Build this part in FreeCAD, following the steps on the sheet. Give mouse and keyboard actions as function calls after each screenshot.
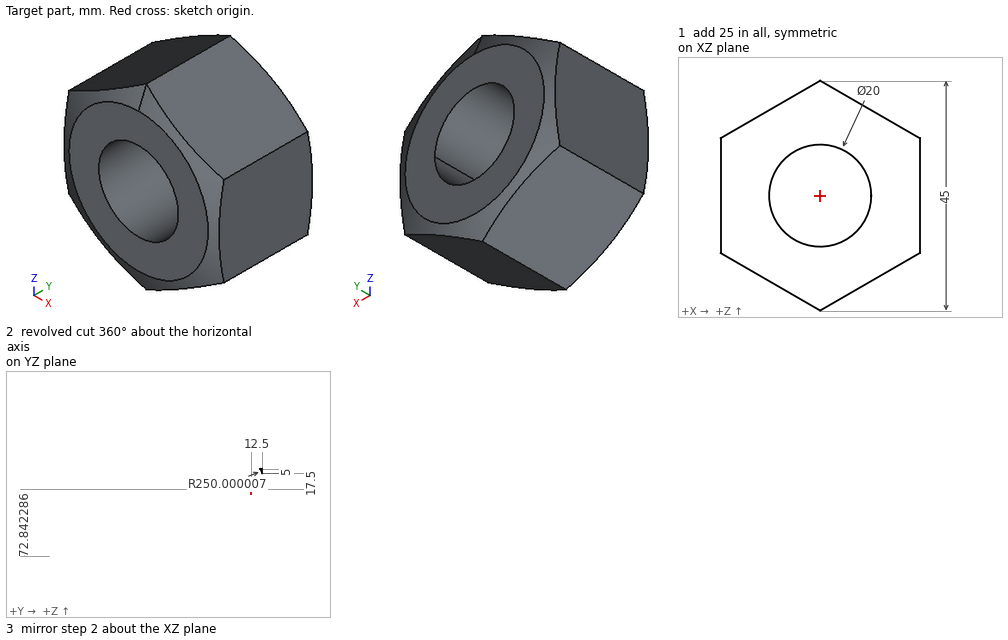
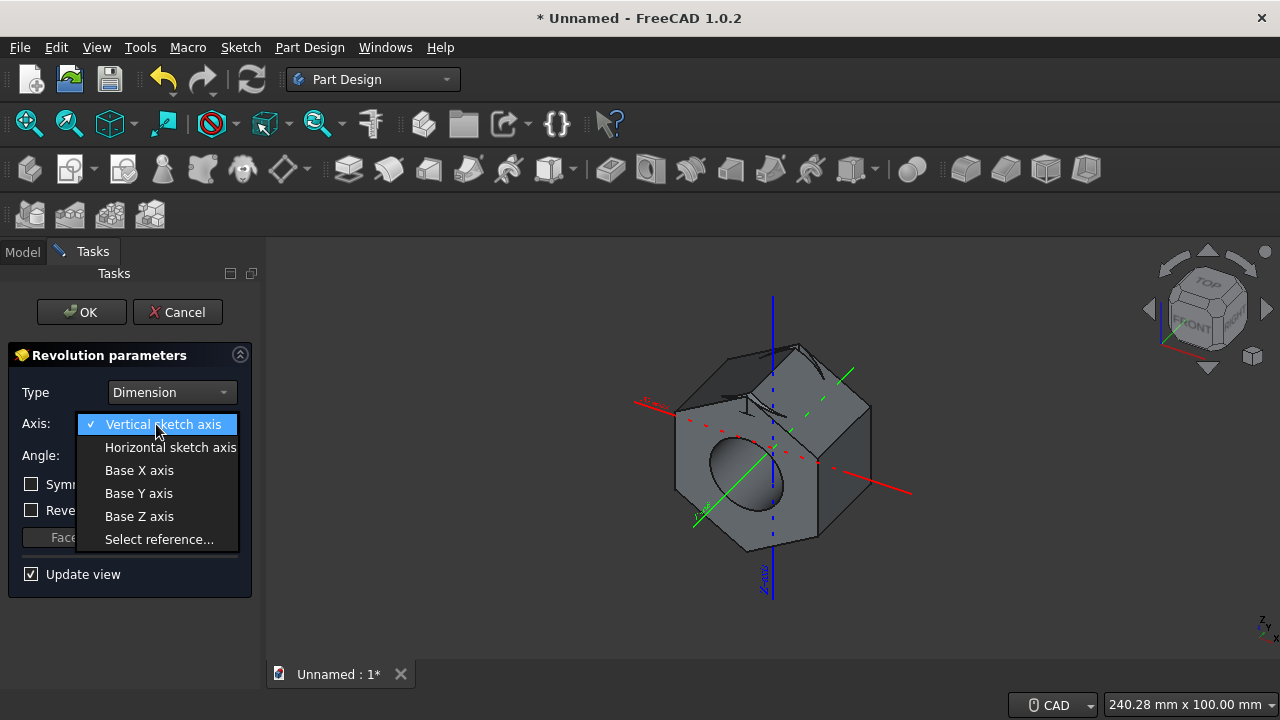
click(156, 448)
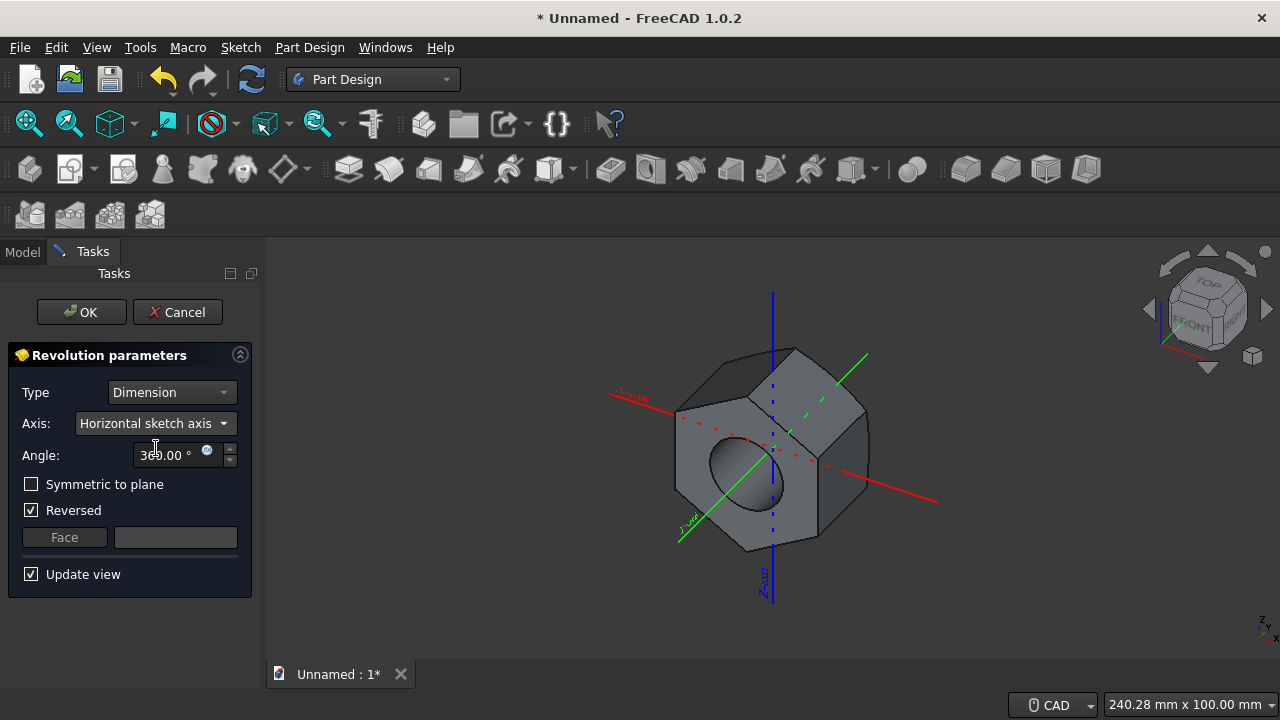
click(82, 312)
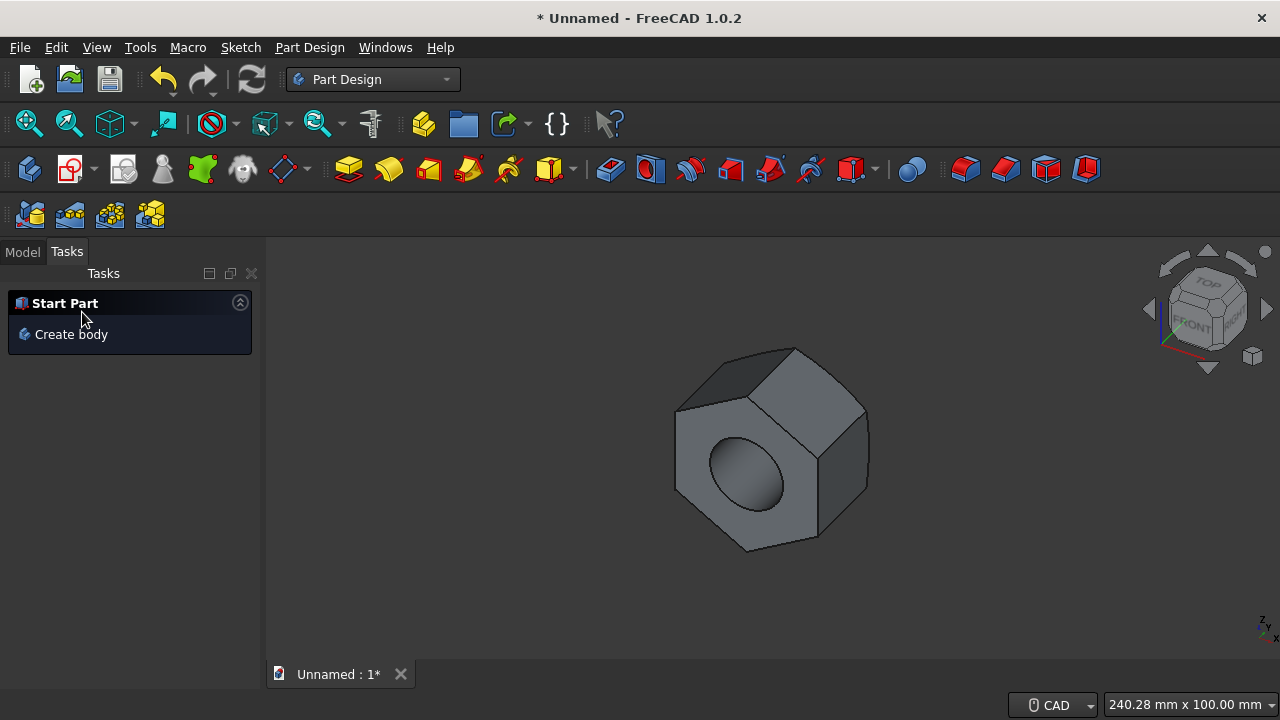
click(23, 251)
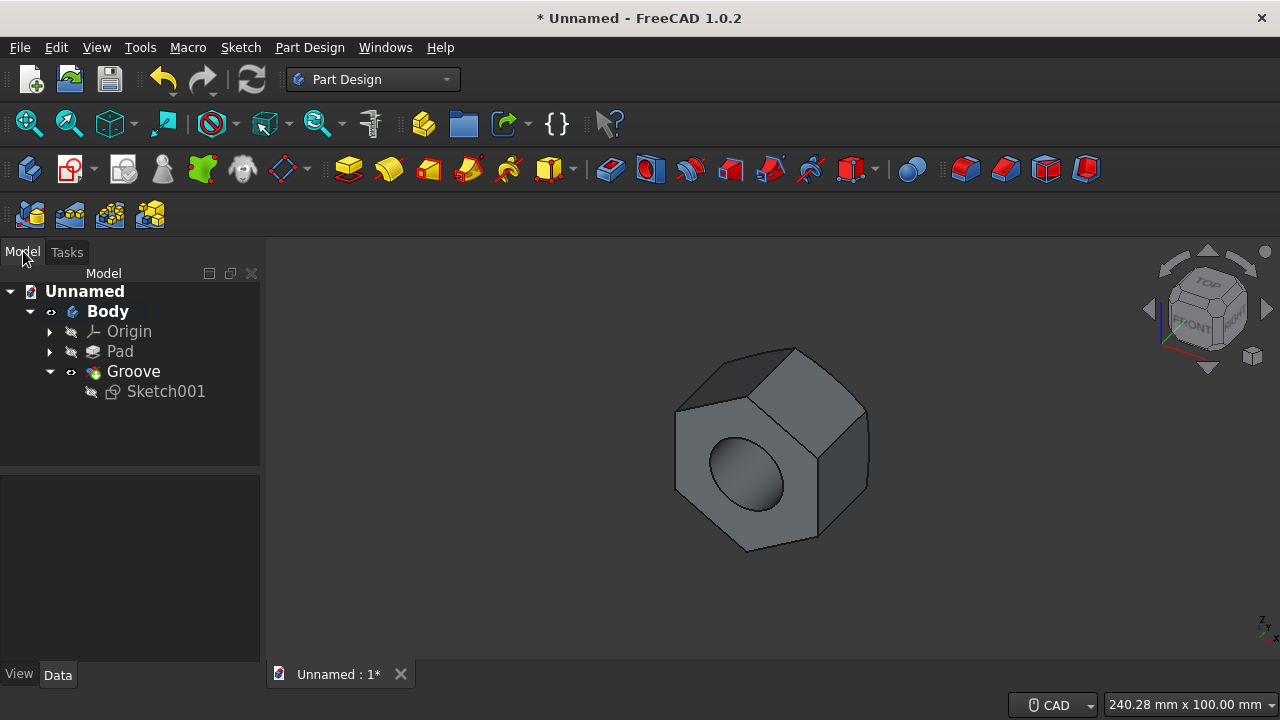
click(116, 372)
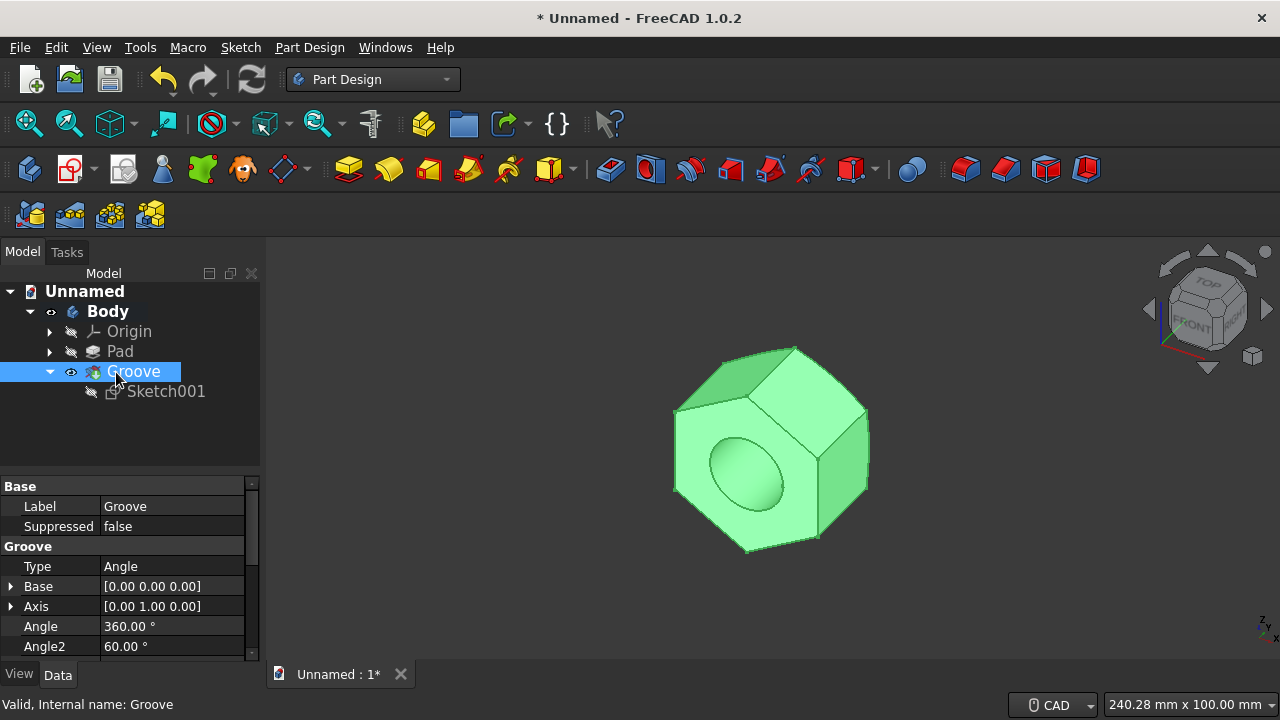
click(30, 214)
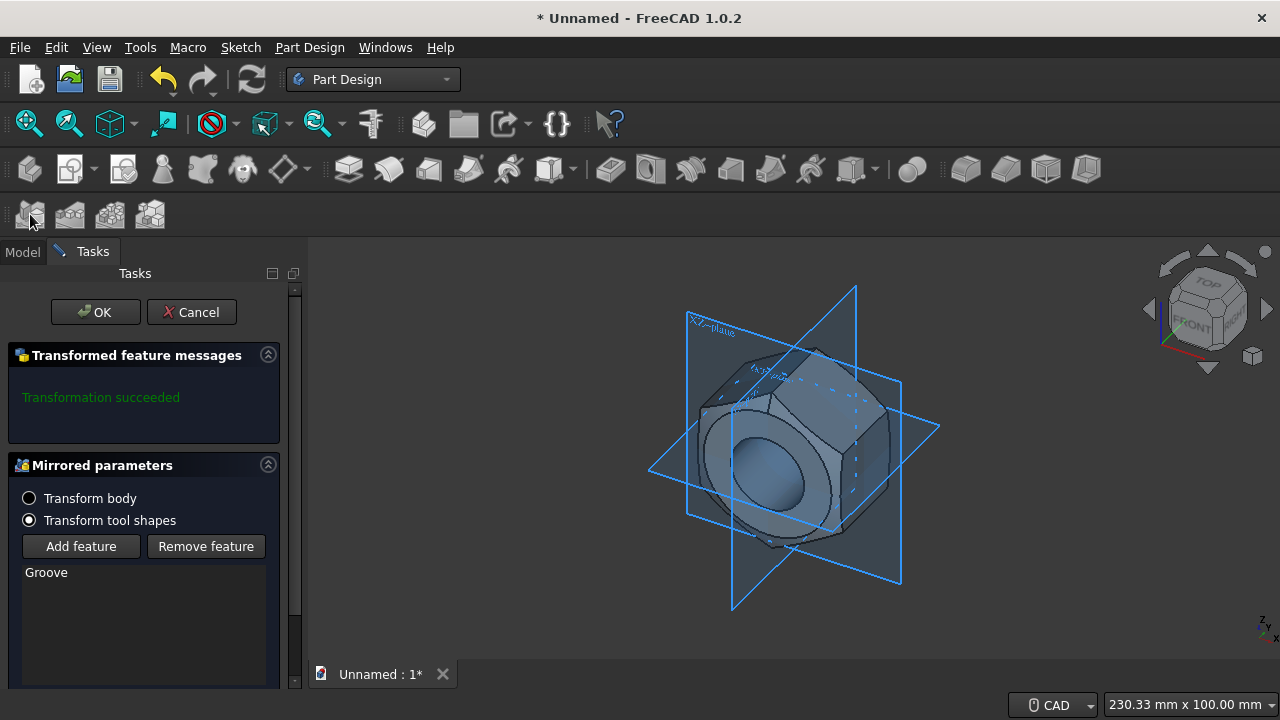
scroll(295, 486, down, 2)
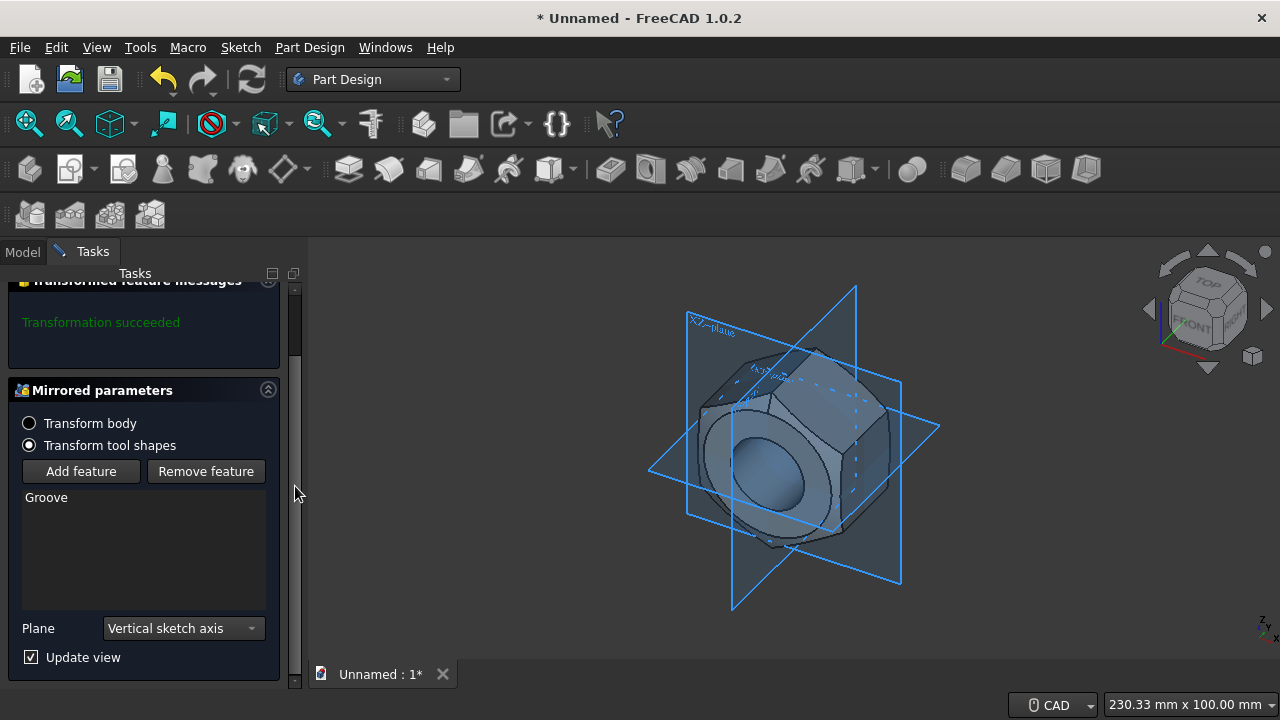
click(184, 628)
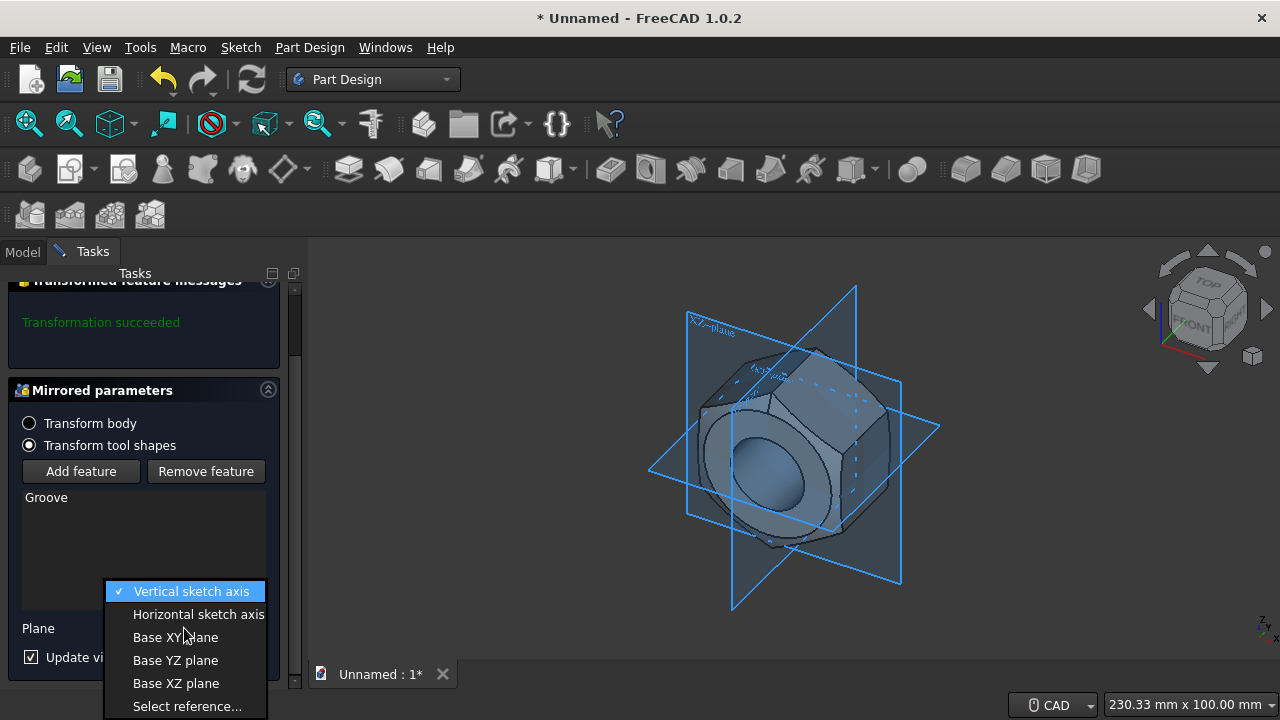
click(184, 684)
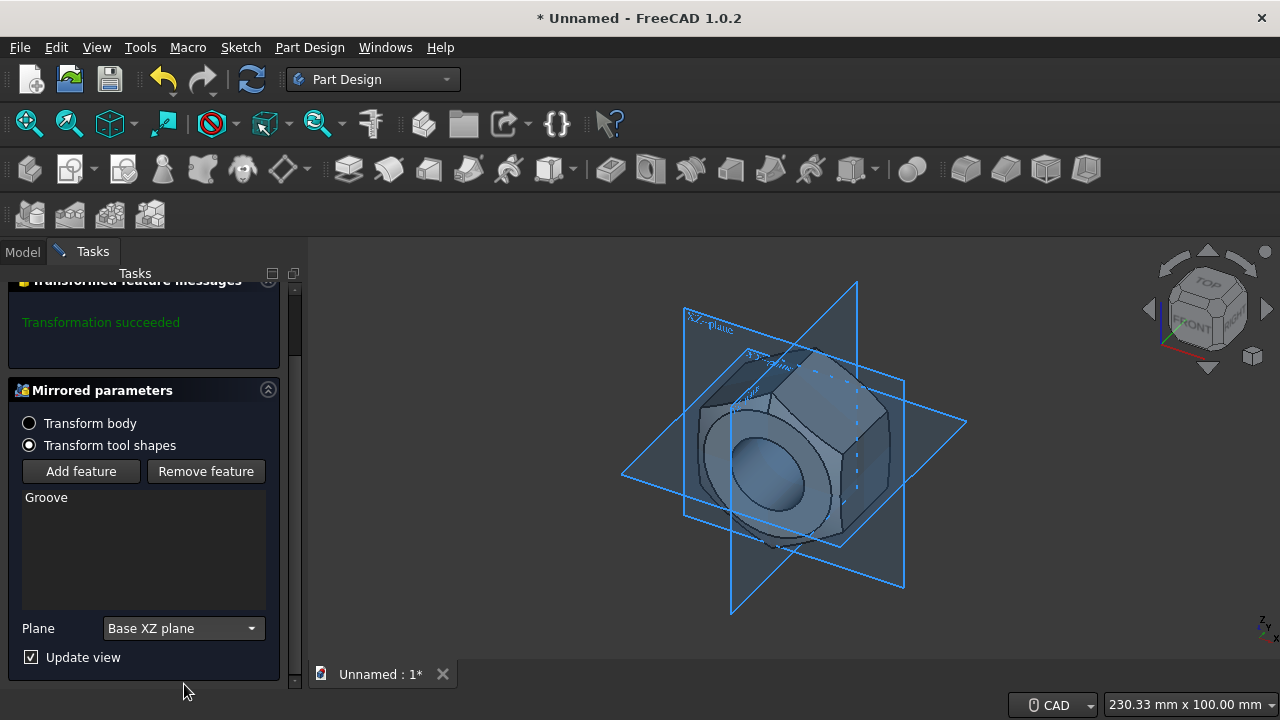
scroll(295, 486, up, 2)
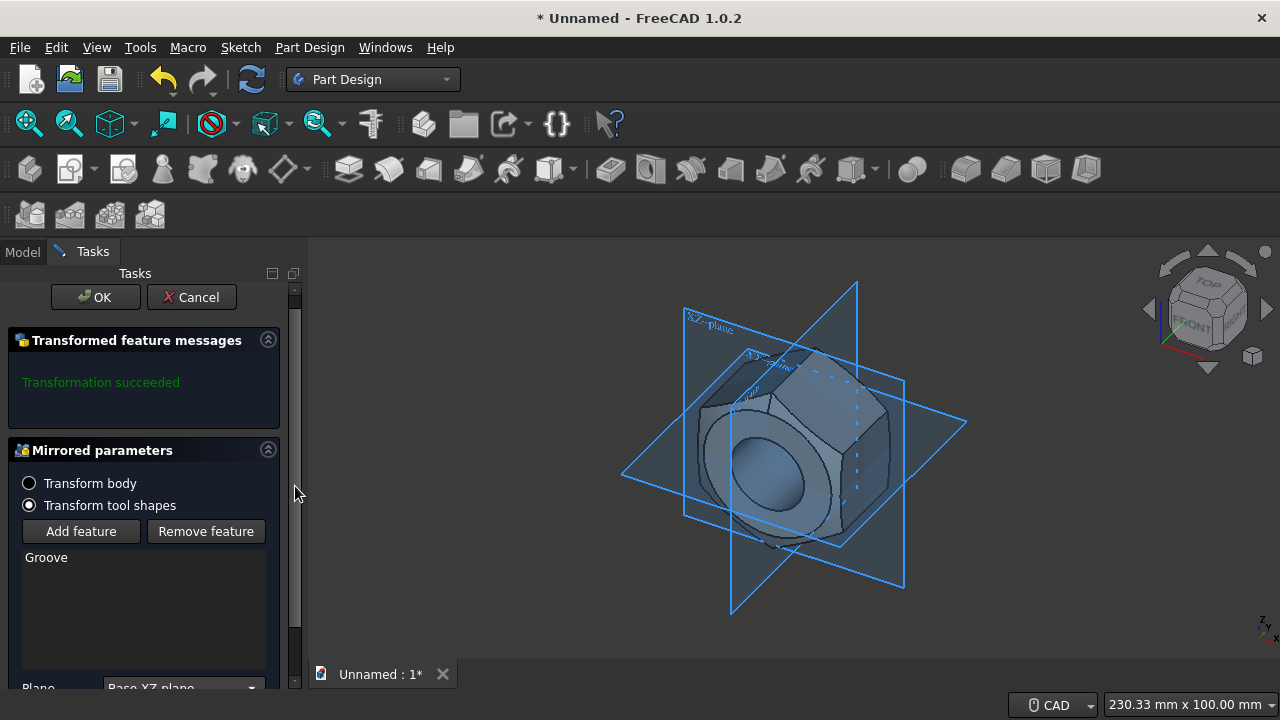
click(96, 312)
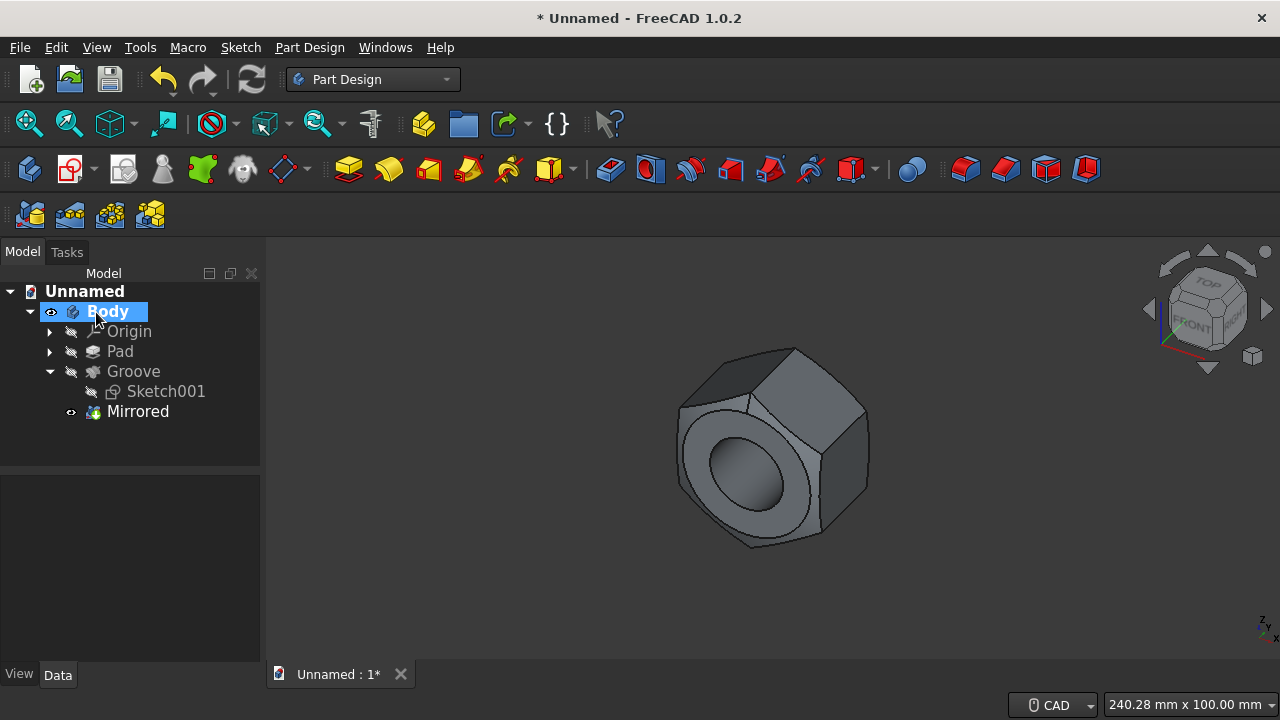
key(0)